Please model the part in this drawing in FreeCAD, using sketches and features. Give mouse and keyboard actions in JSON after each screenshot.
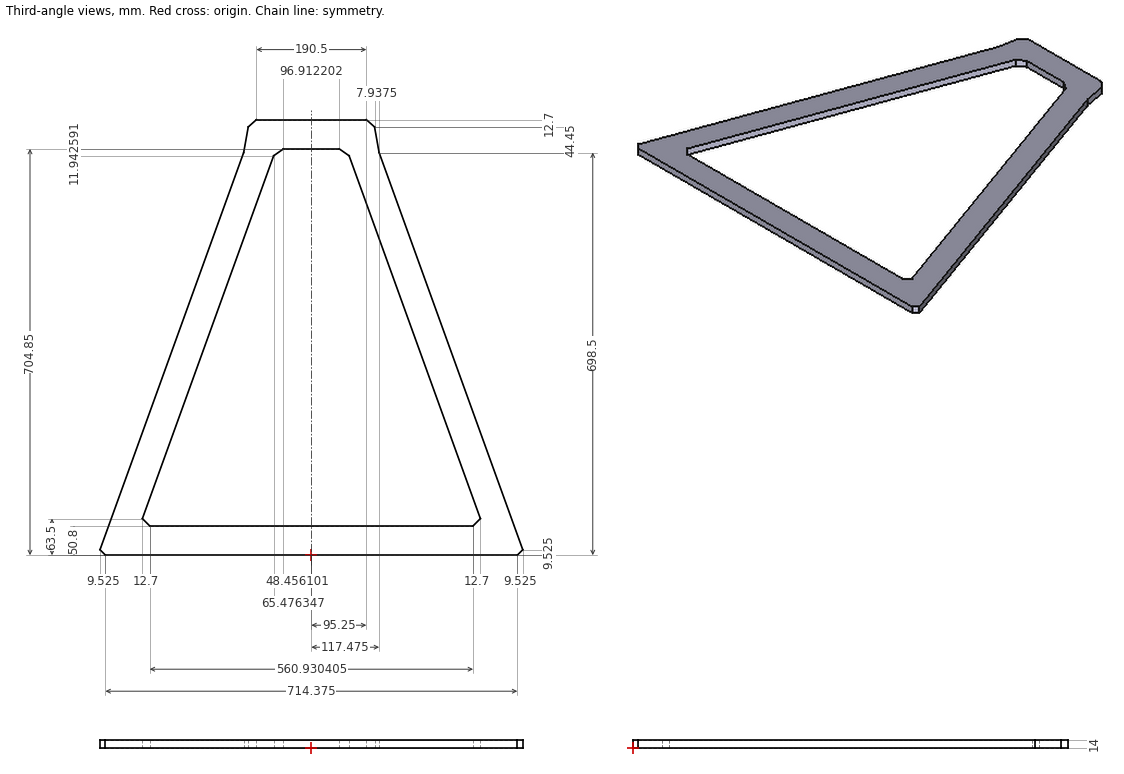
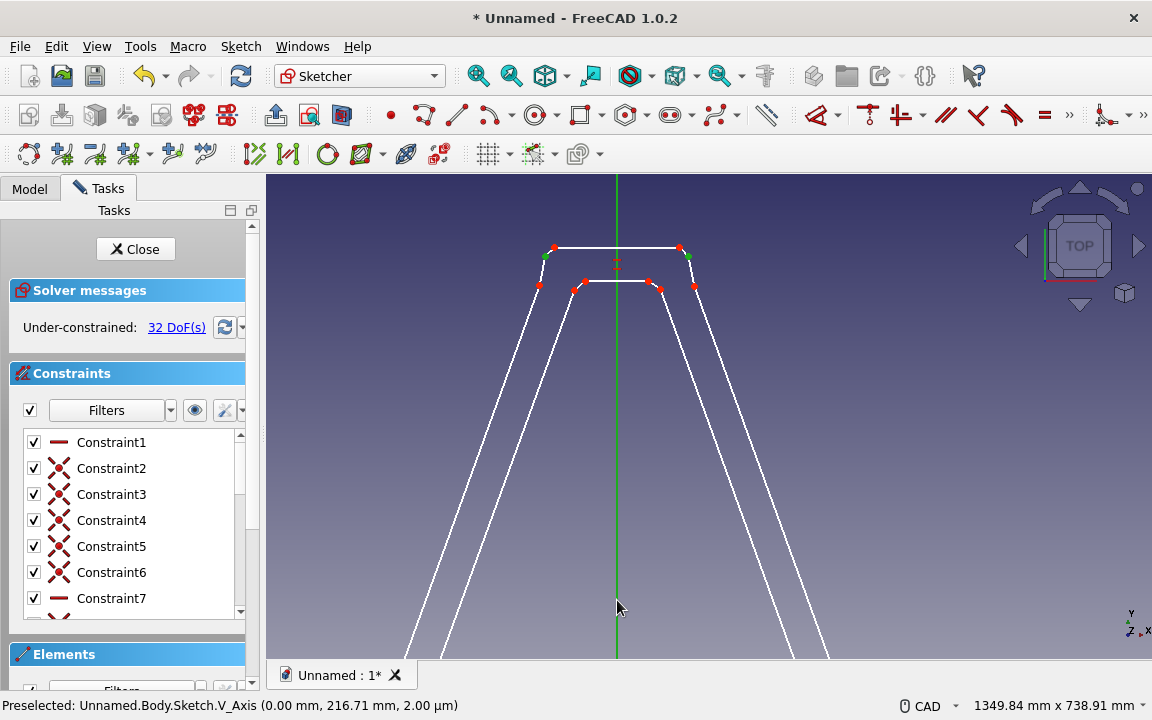
{"action": "key", "text": "s"}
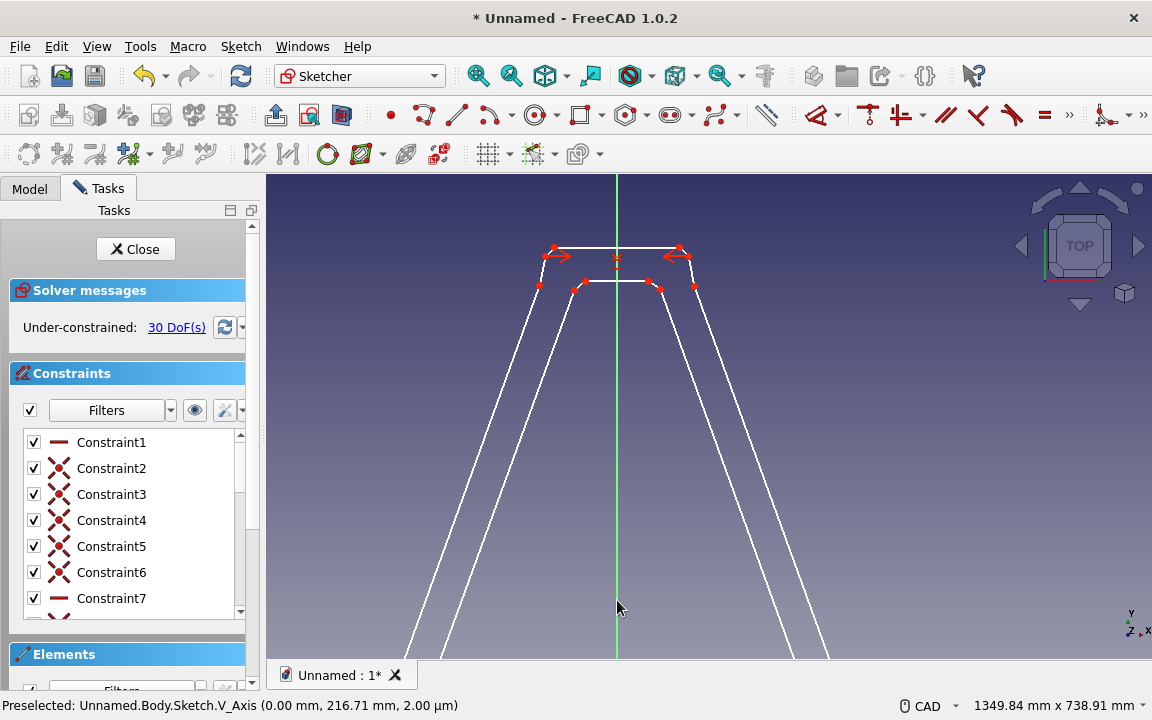
{"action": "left_click", "coordinate": [694, 286]}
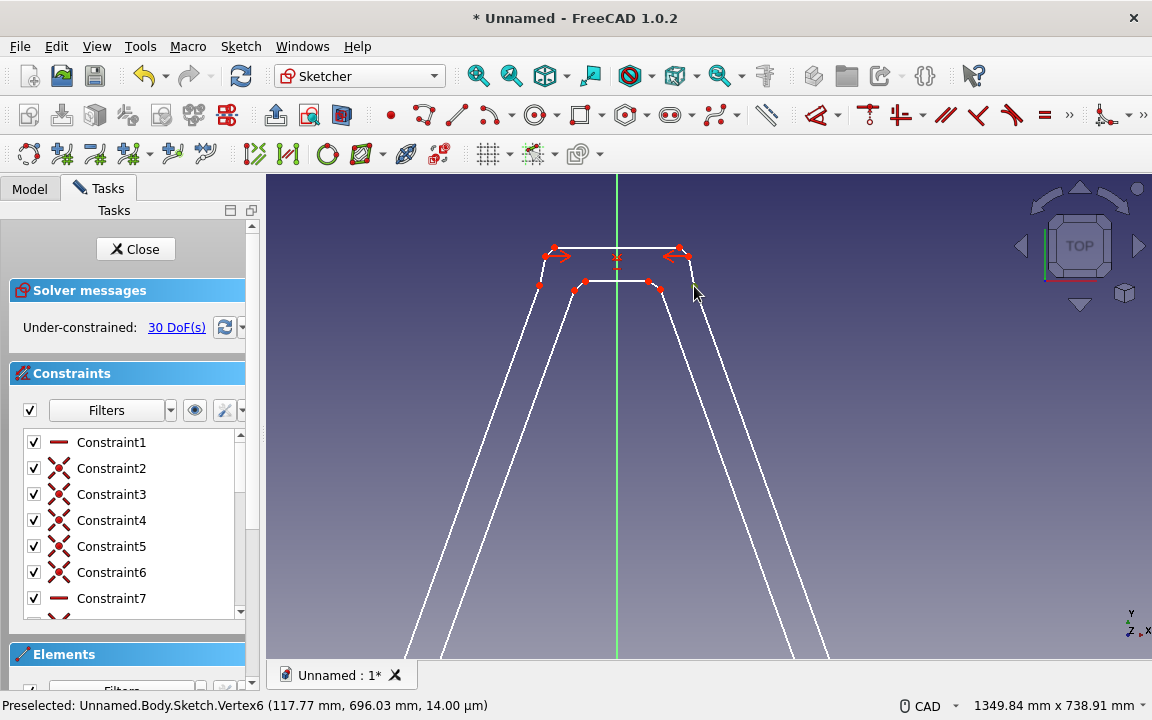
{"action": "left_click", "coordinate": [540, 285]}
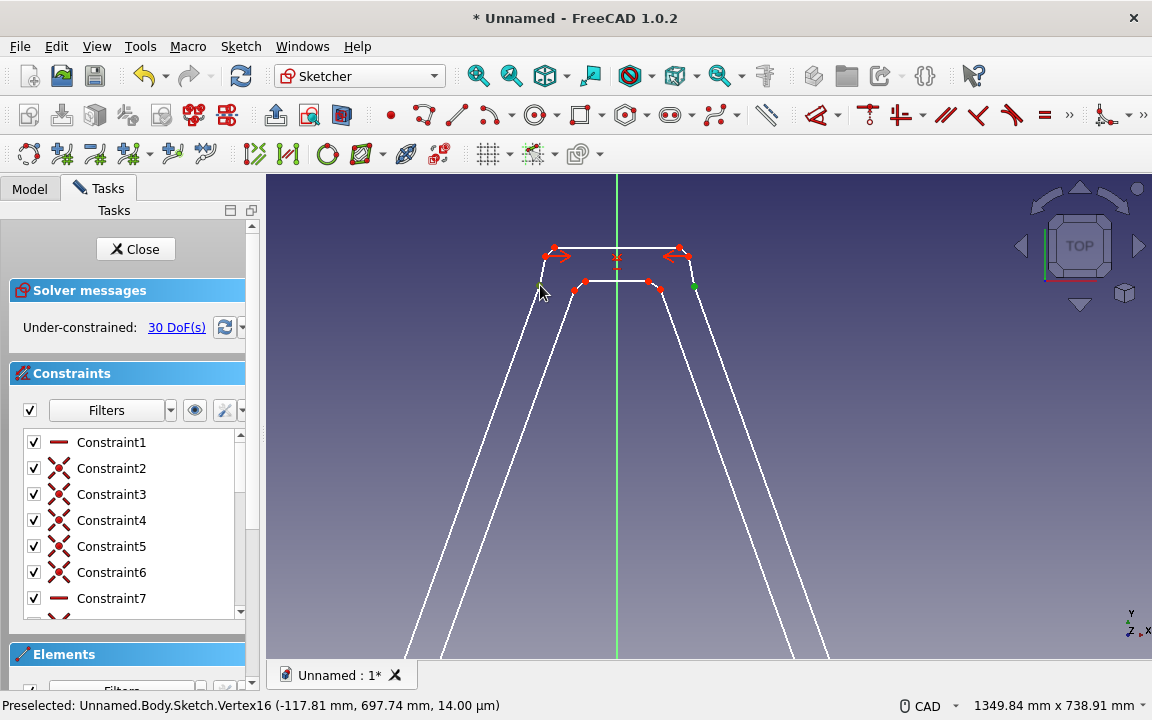
{"action": "left_click", "coordinate": [617, 600]}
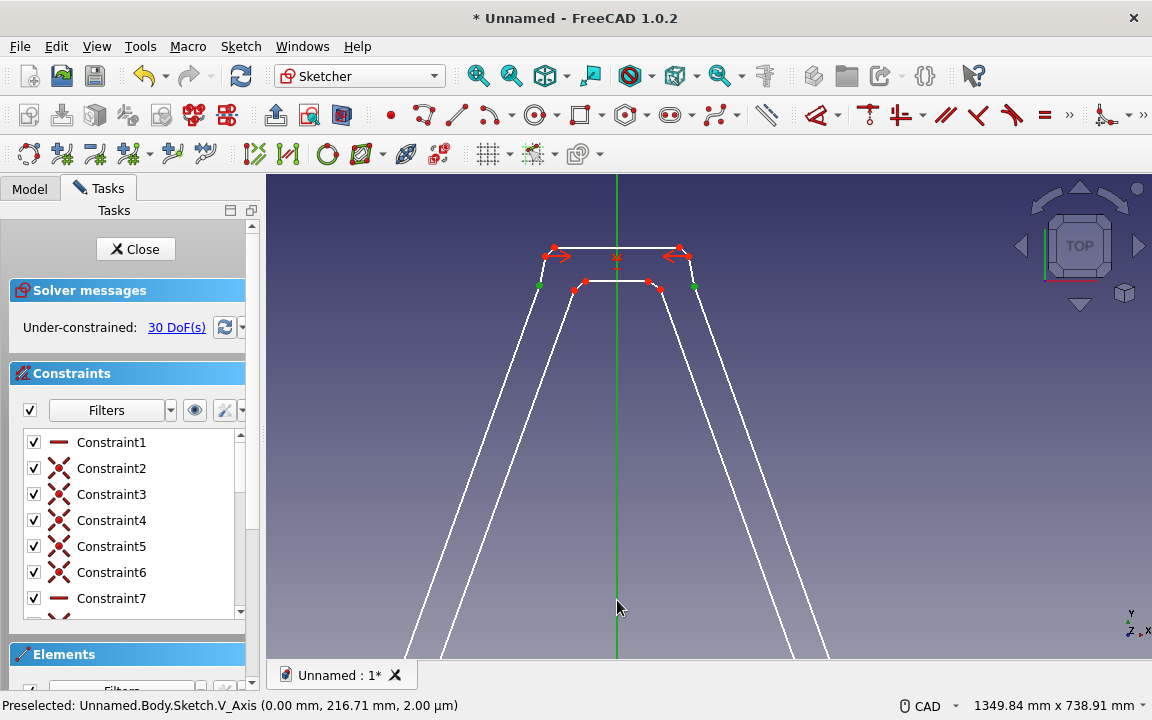
{"action": "key", "text": "s"}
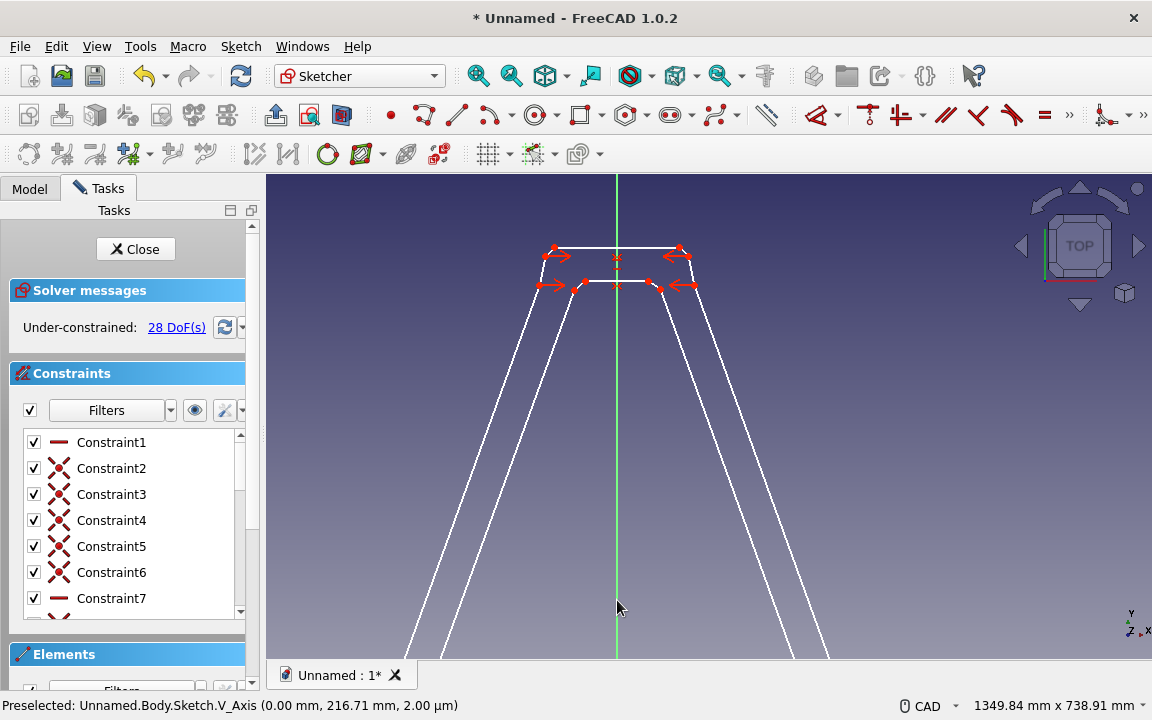
{"action": "scroll", "coordinate": [688, 256], "scroll_direction": "down", "scroll_amount": 2}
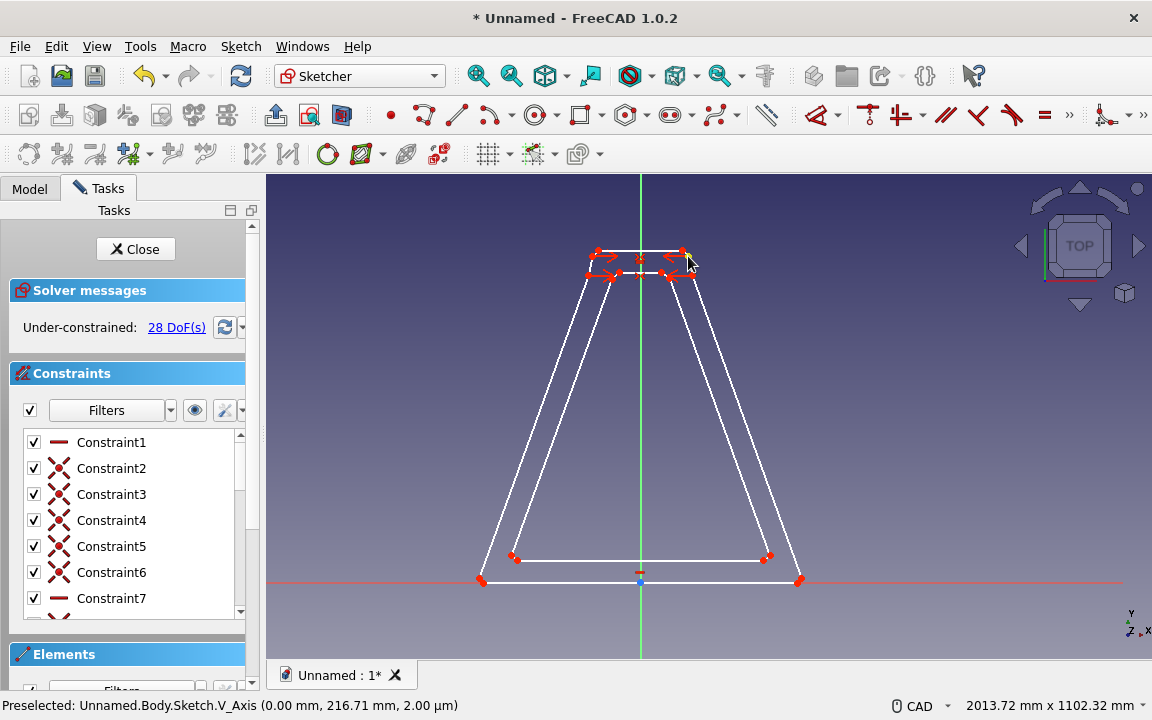
{"action": "scroll", "coordinate": [802, 579], "scroll_direction": "up", "scroll_amount": 4}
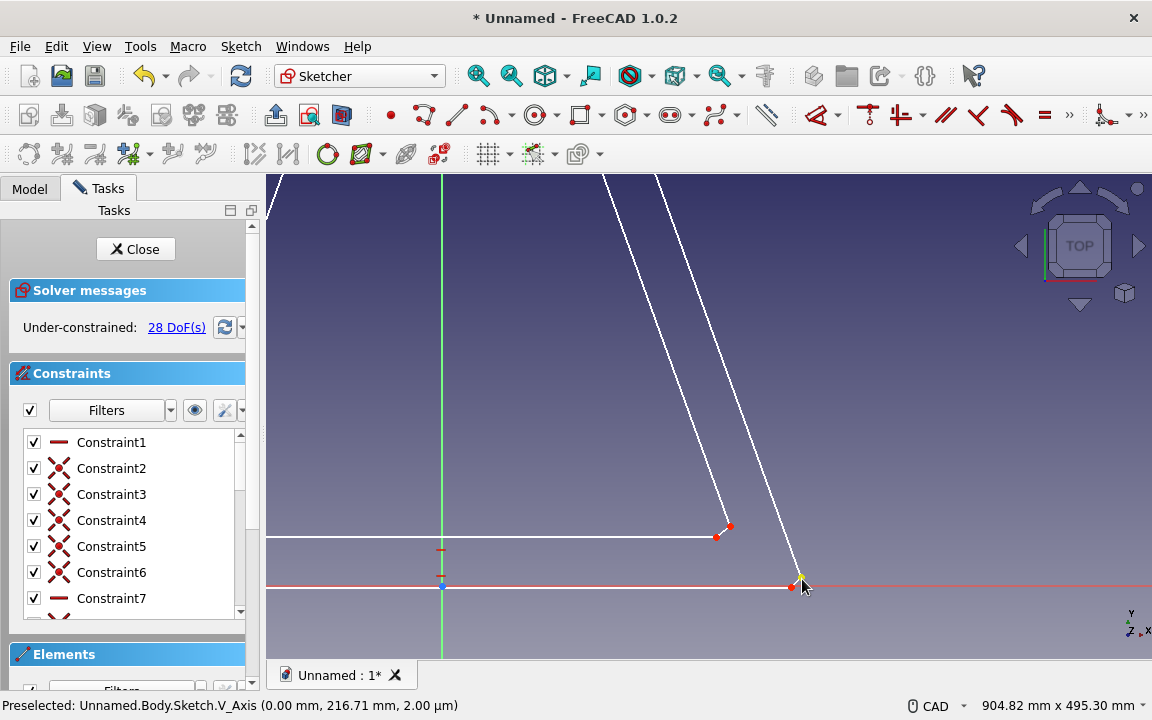
{"action": "left_click", "coordinate": [801, 578]}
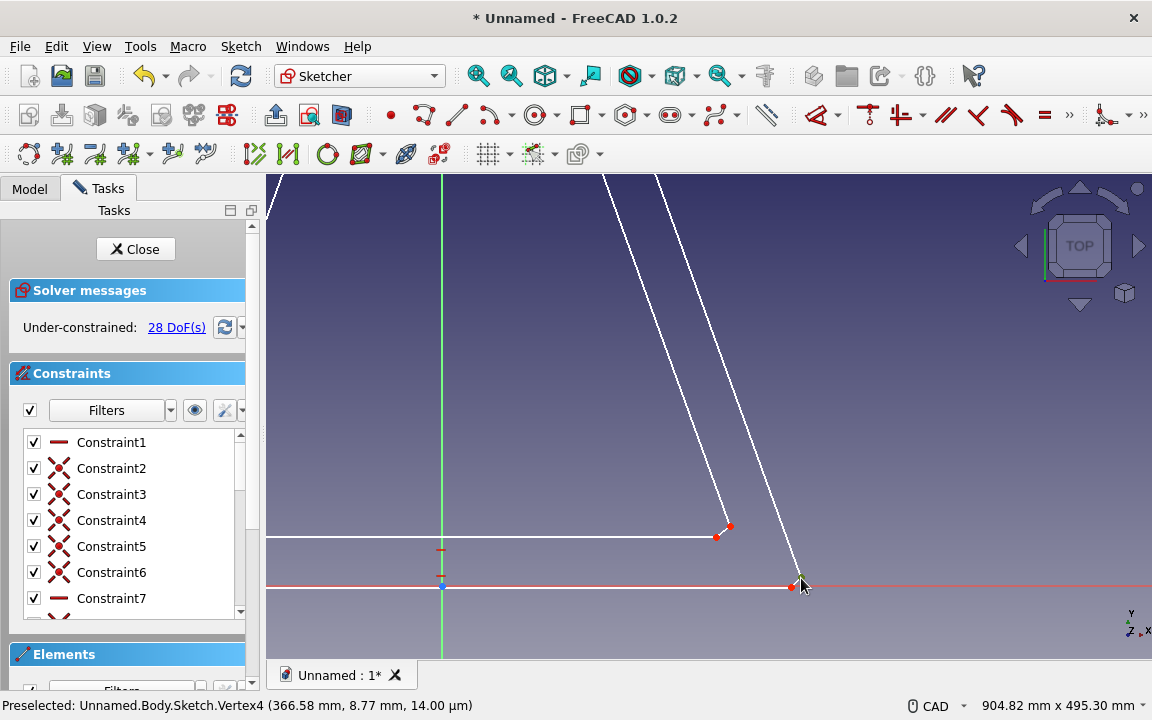
{"action": "scroll", "coordinate": [802, 580], "scroll_direction": "down", "scroll_amount": 4}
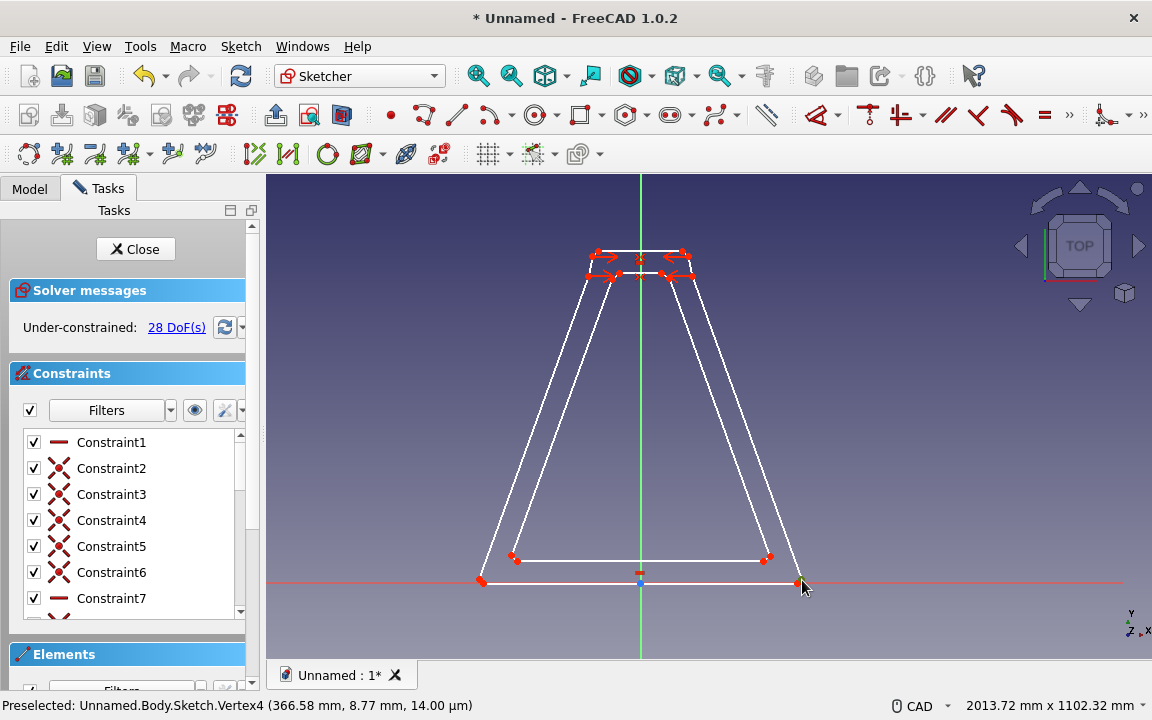
{"action": "scroll", "coordinate": [479, 579], "scroll_direction": "up", "scroll_amount": 4}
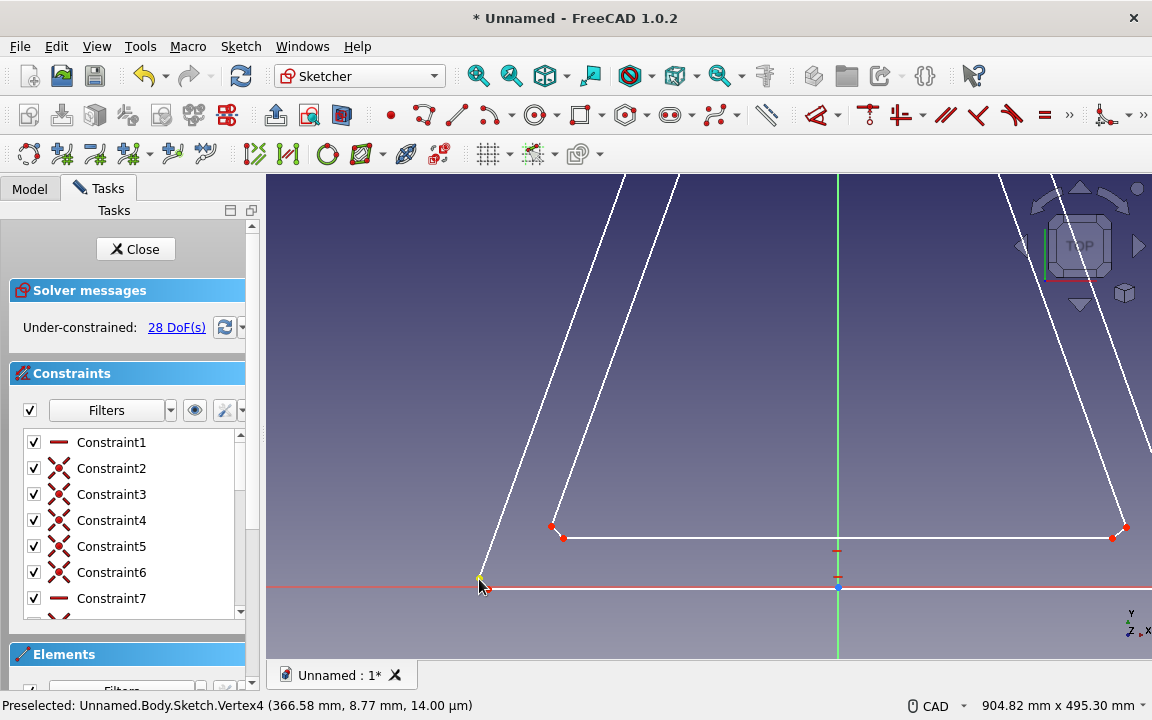
{"action": "left_click", "coordinate": [479, 578]}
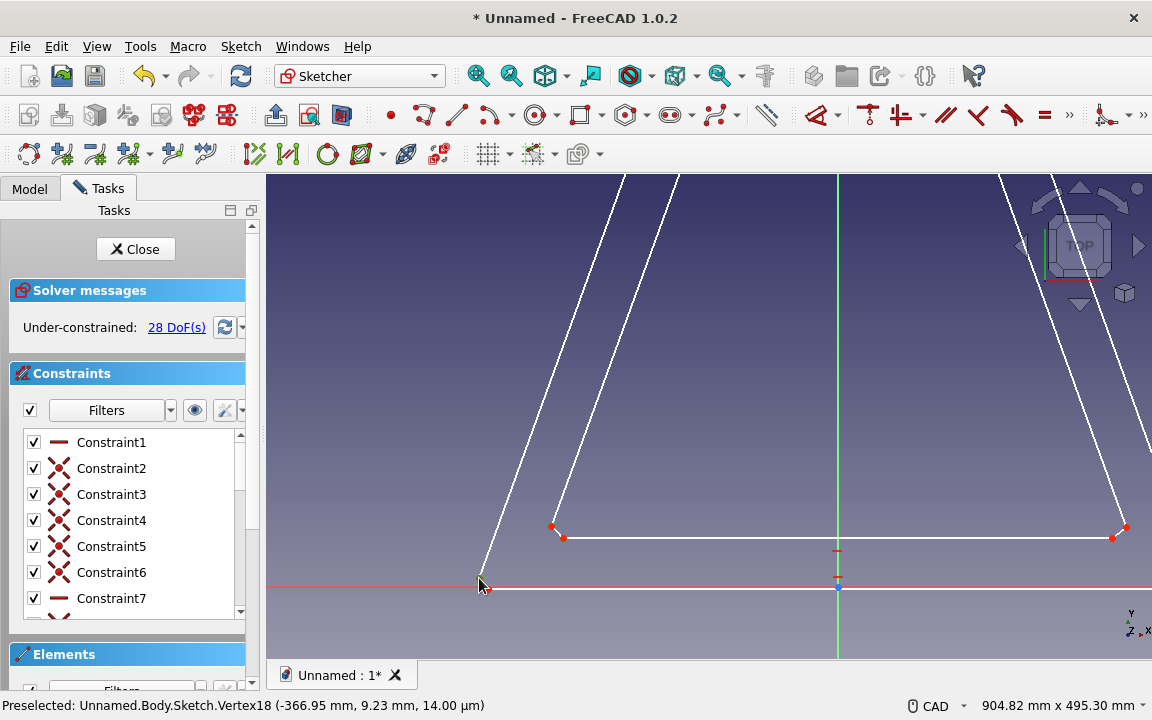
{"action": "left_click", "coordinate": [838, 478]}